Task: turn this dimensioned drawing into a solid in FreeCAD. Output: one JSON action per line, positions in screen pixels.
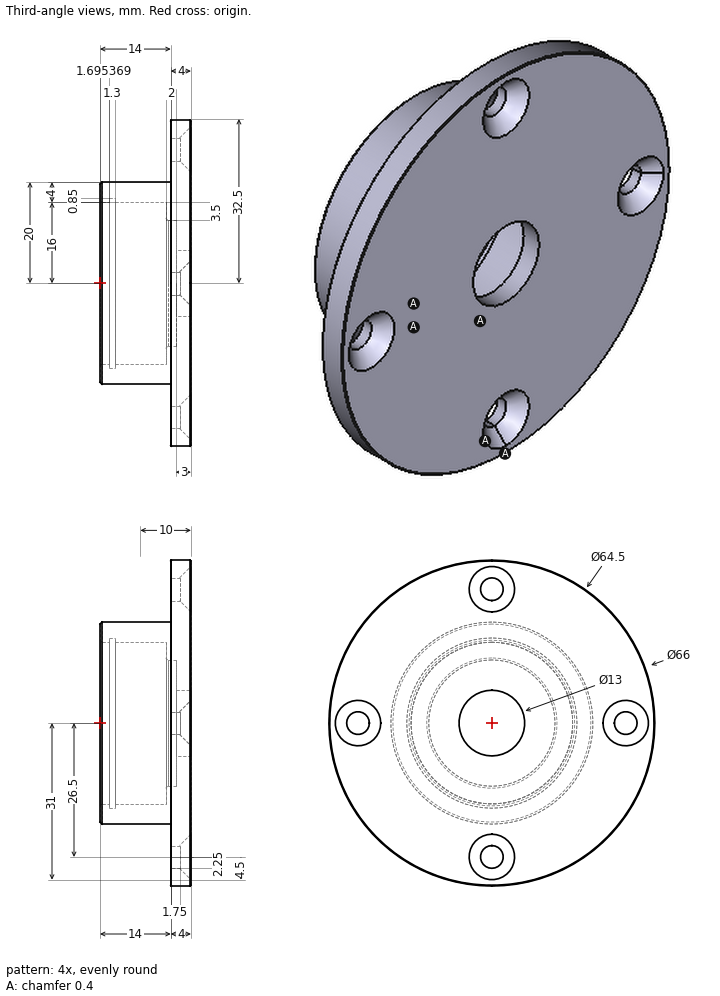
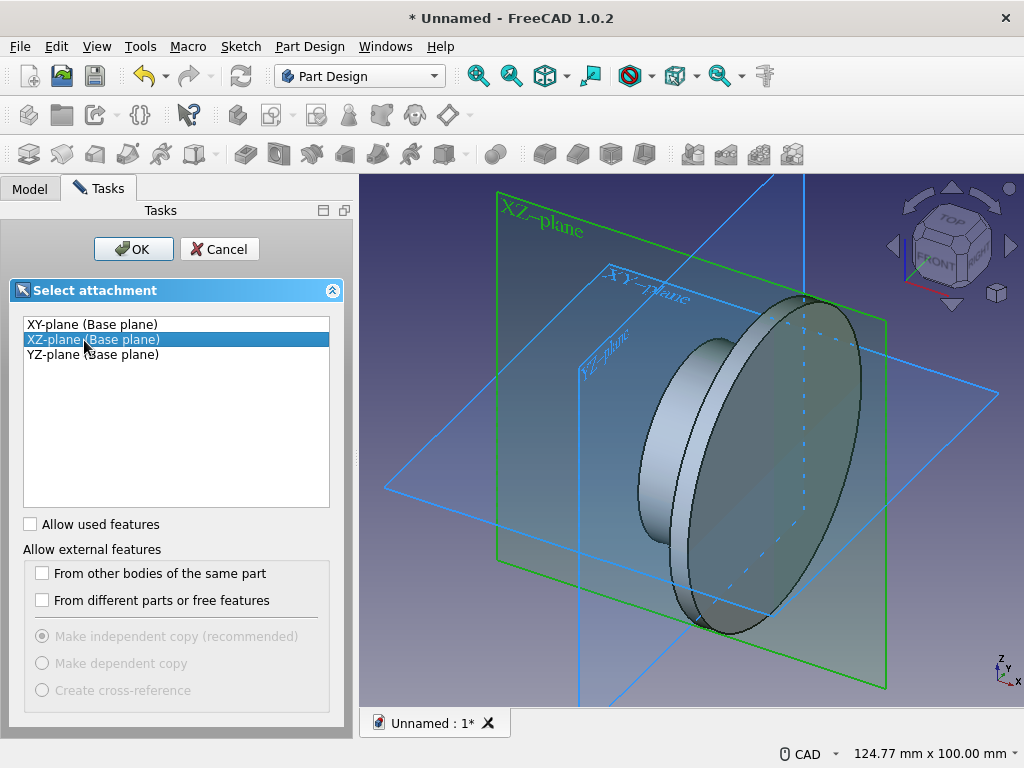
{"action": "left_click", "coordinate": [134, 249]}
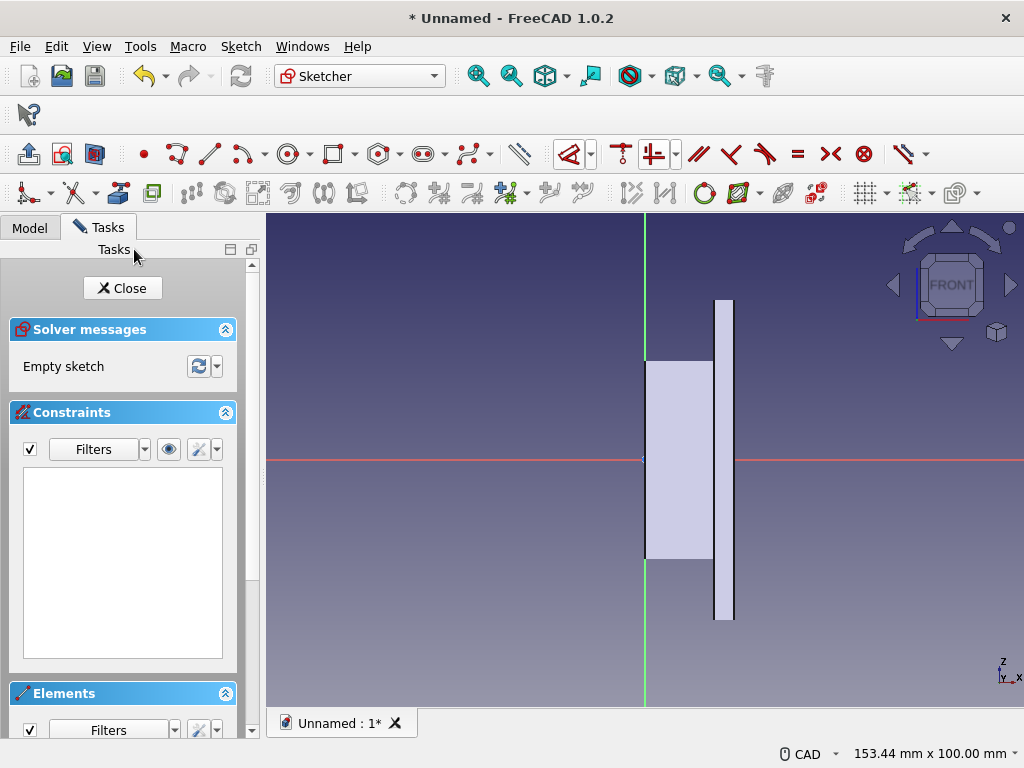
{"action": "left_click", "coordinate": [95, 154]}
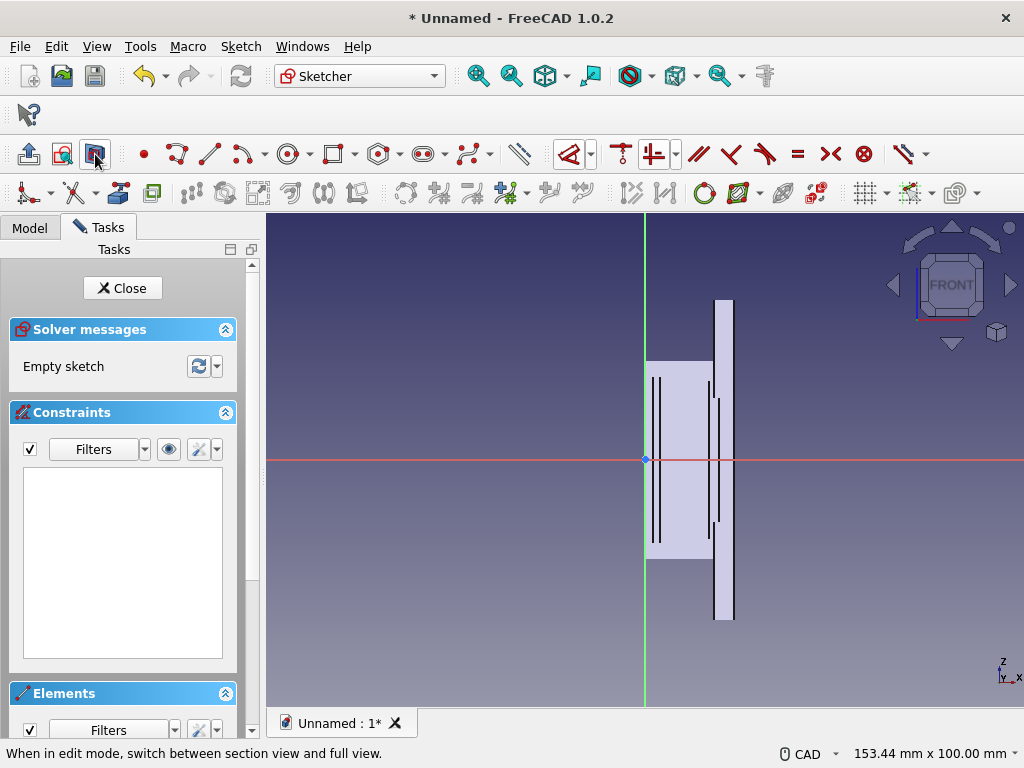
{"action": "scroll", "coordinate": [740, 613], "scroll_direction": "up", "scroll_amount": 13}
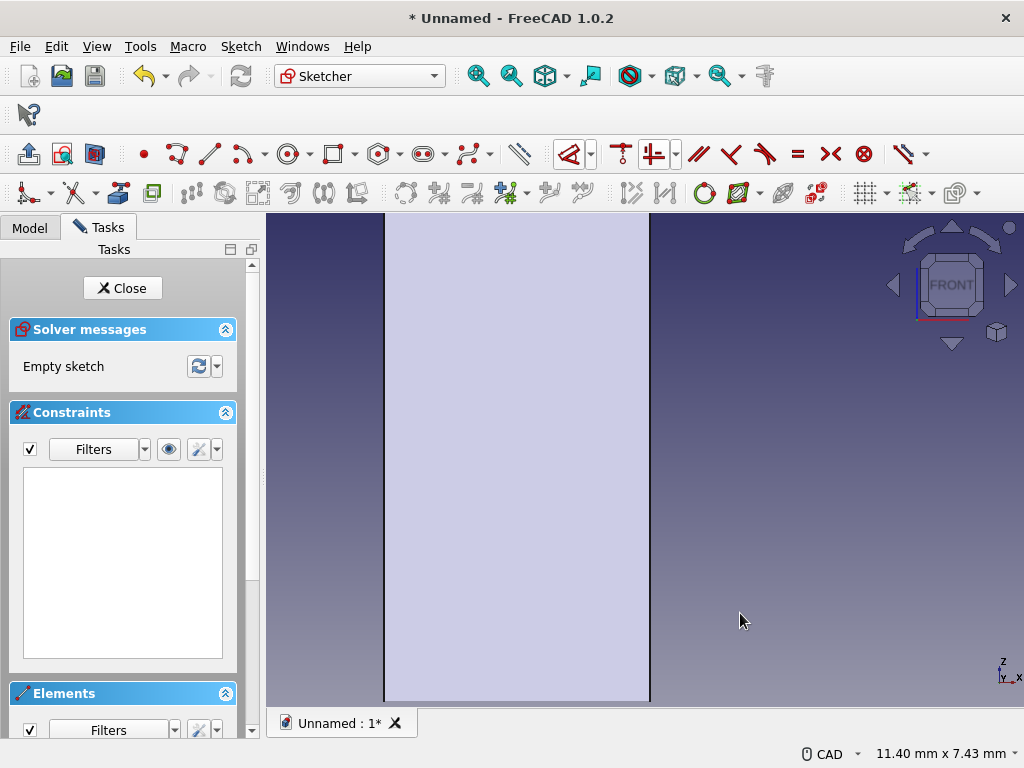
{"action": "left_click", "coordinate": [177, 154]}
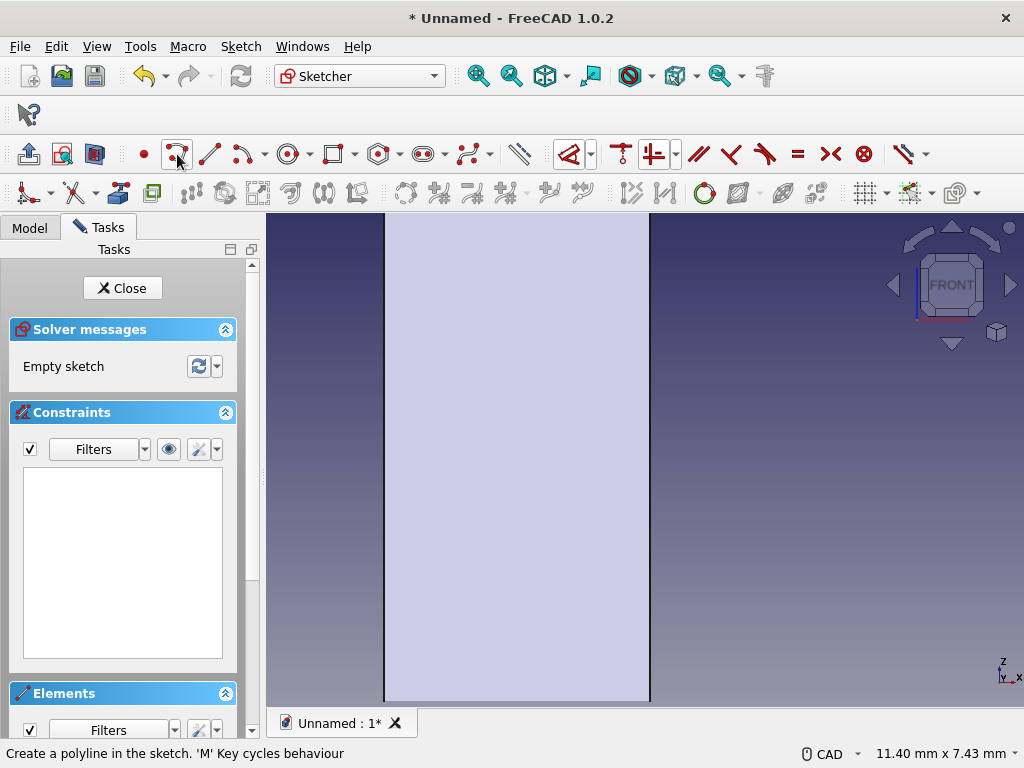
{"action": "left_click", "coordinate": [384, 305]}
{"action": "left_click", "coordinate": [650, 305]}
{"action": "left_click", "coordinate": [650, 605]}
{"action": "left_click", "coordinate": [501, 455]}
{"action": "left_click", "coordinate": [384, 455]}
{"action": "left_click", "coordinate": [384, 306]}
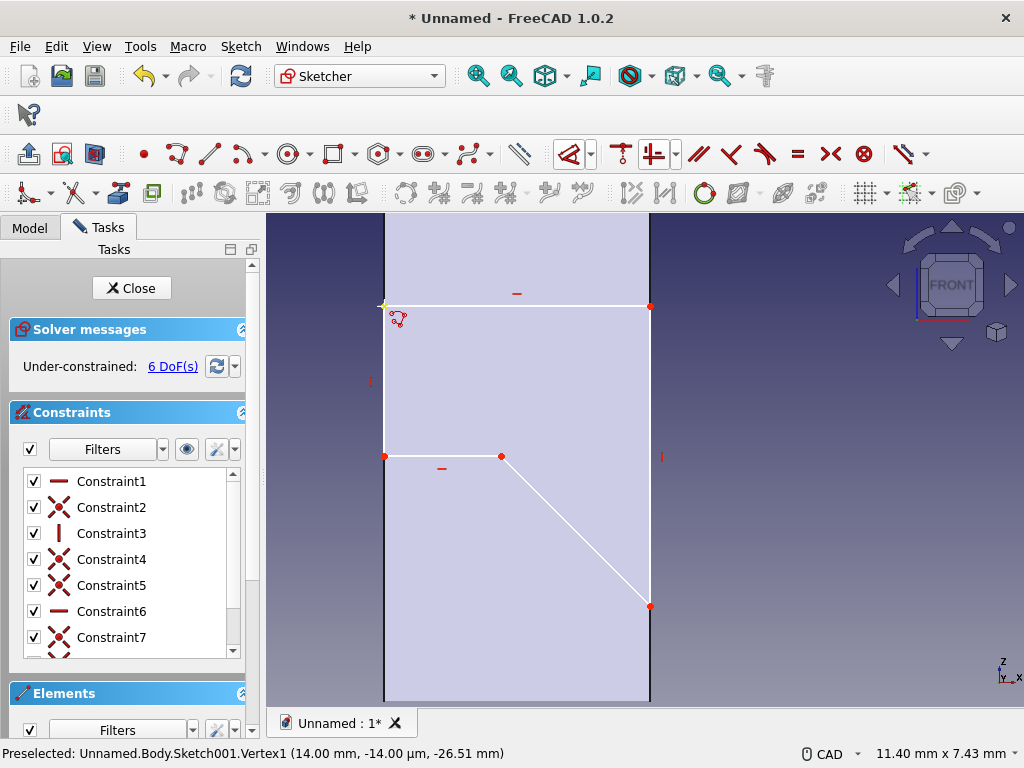
{"action": "left_click", "coordinate": [210, 154]}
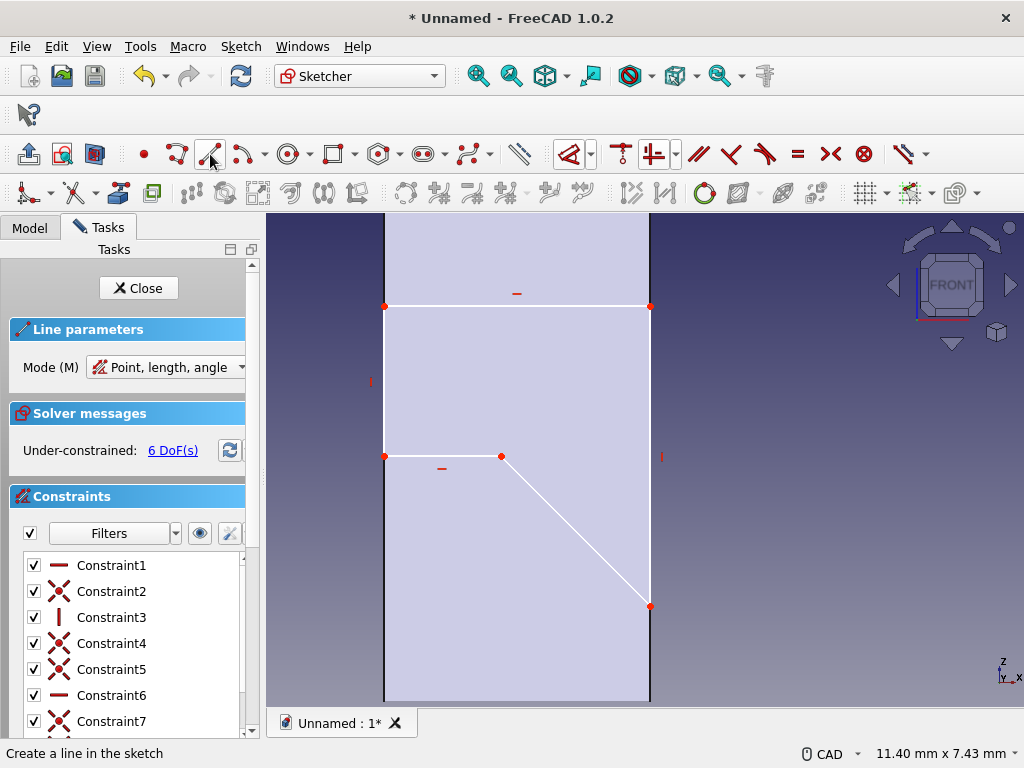
{"action": "left_click", "coordinate": [677, 305]}
{"action": "left_click", "coordinate": [757, 305]}
{"action": "key", "text": "Escape"}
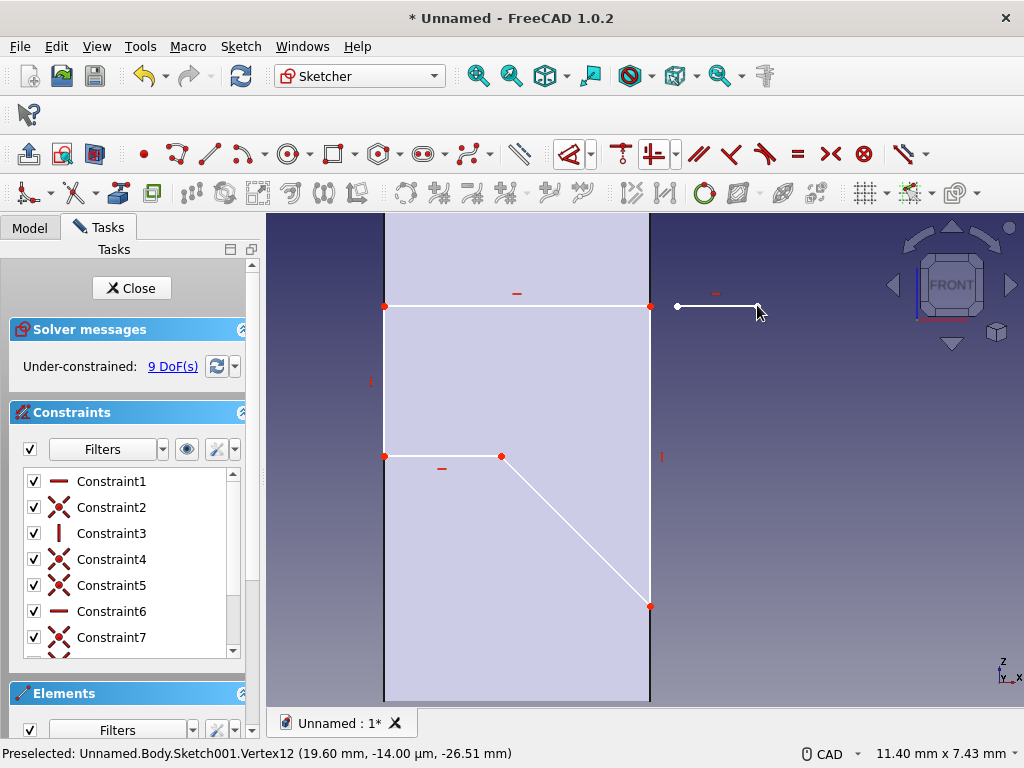
{"action": "left_click", "coordinate": [701, 306]}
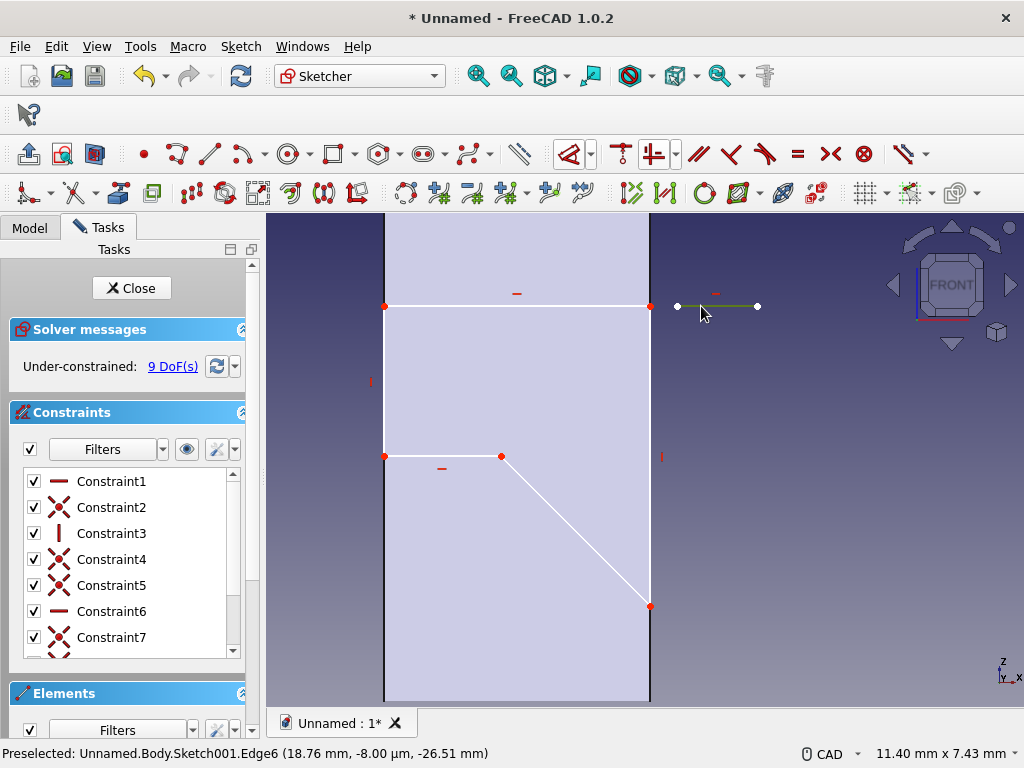
{"action": "left_click", "coordinate": [520, 154]}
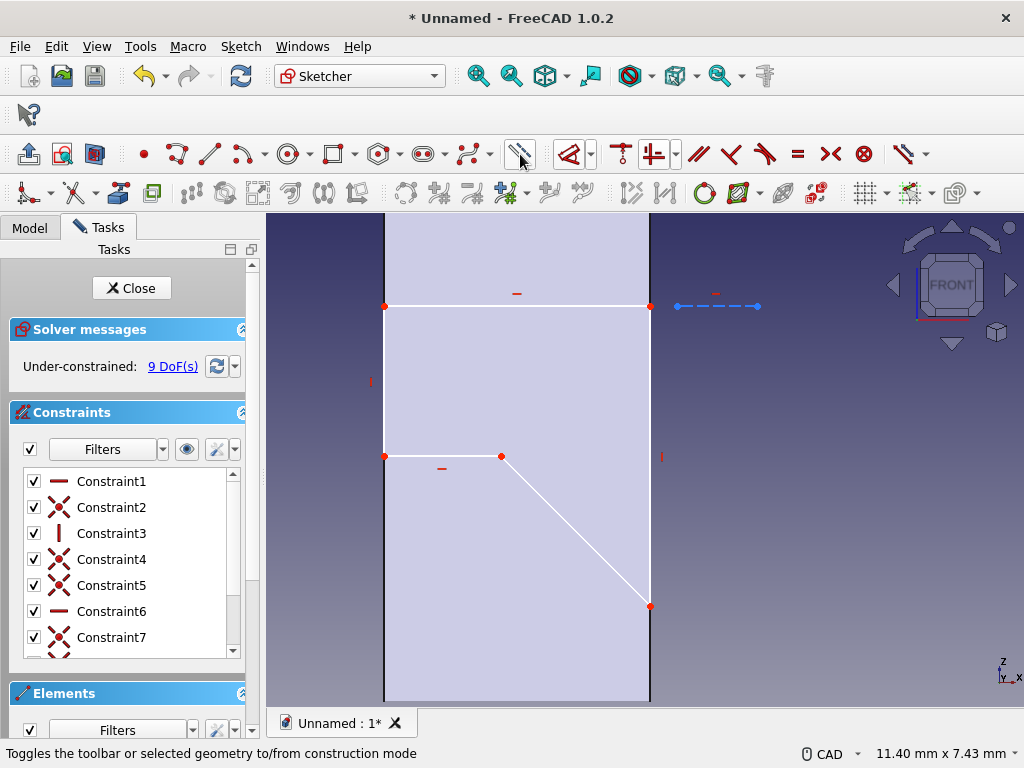
{"action": "left_click", "coordinate": [464, 306]}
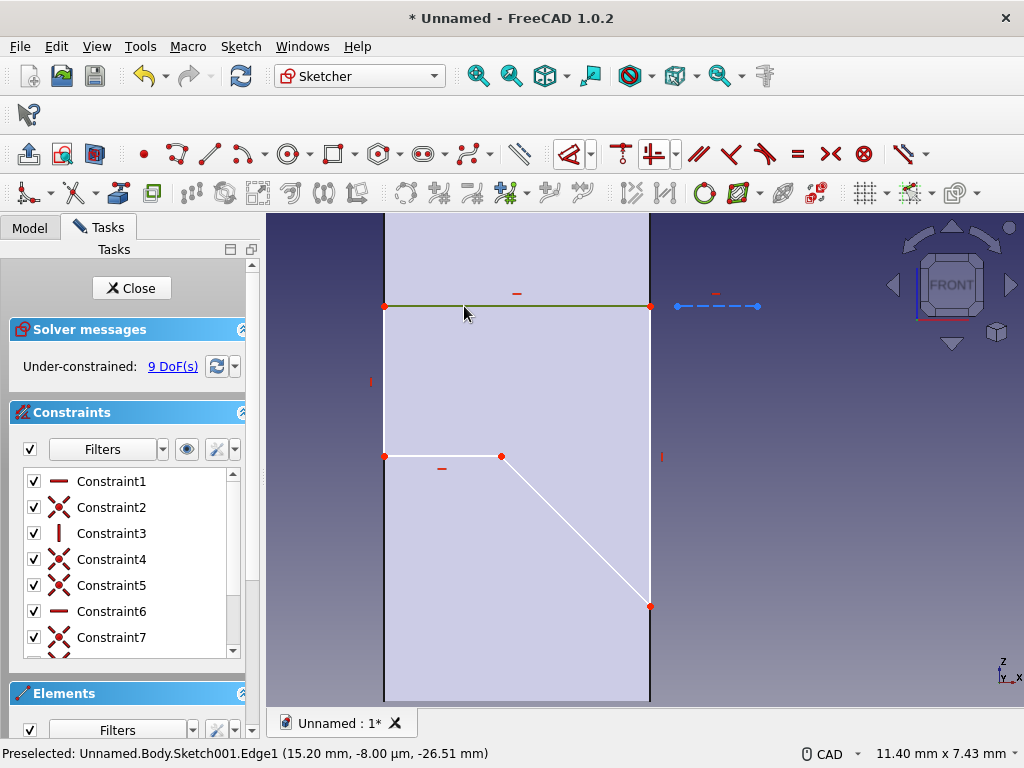
{"action": "left_click", "coordinate": [590, 154]}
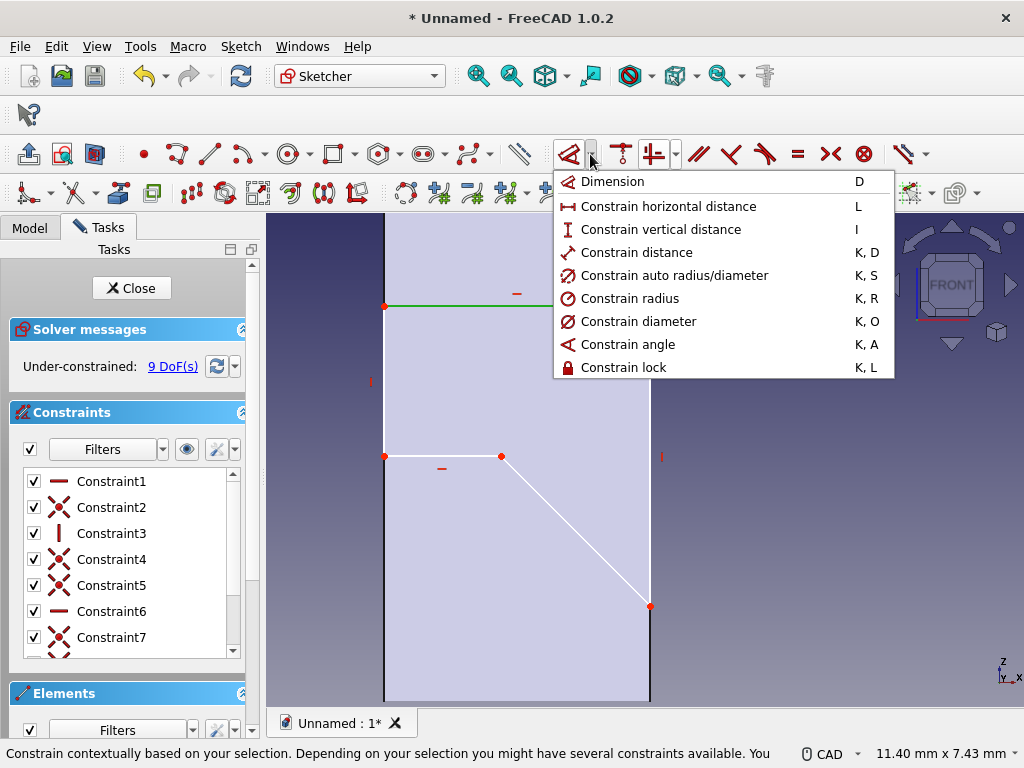
{"action": "left_click", "coordinate": [724, 206]}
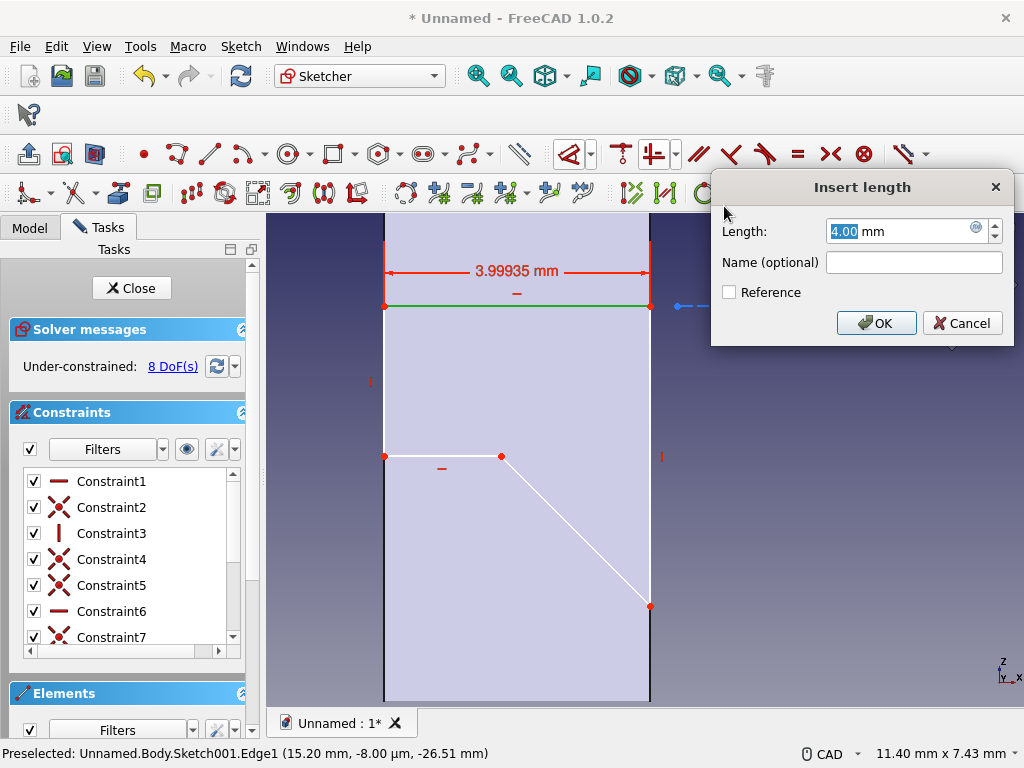
{"action": "type", "text": "4"}
{"action": "key", "text": "Return"}